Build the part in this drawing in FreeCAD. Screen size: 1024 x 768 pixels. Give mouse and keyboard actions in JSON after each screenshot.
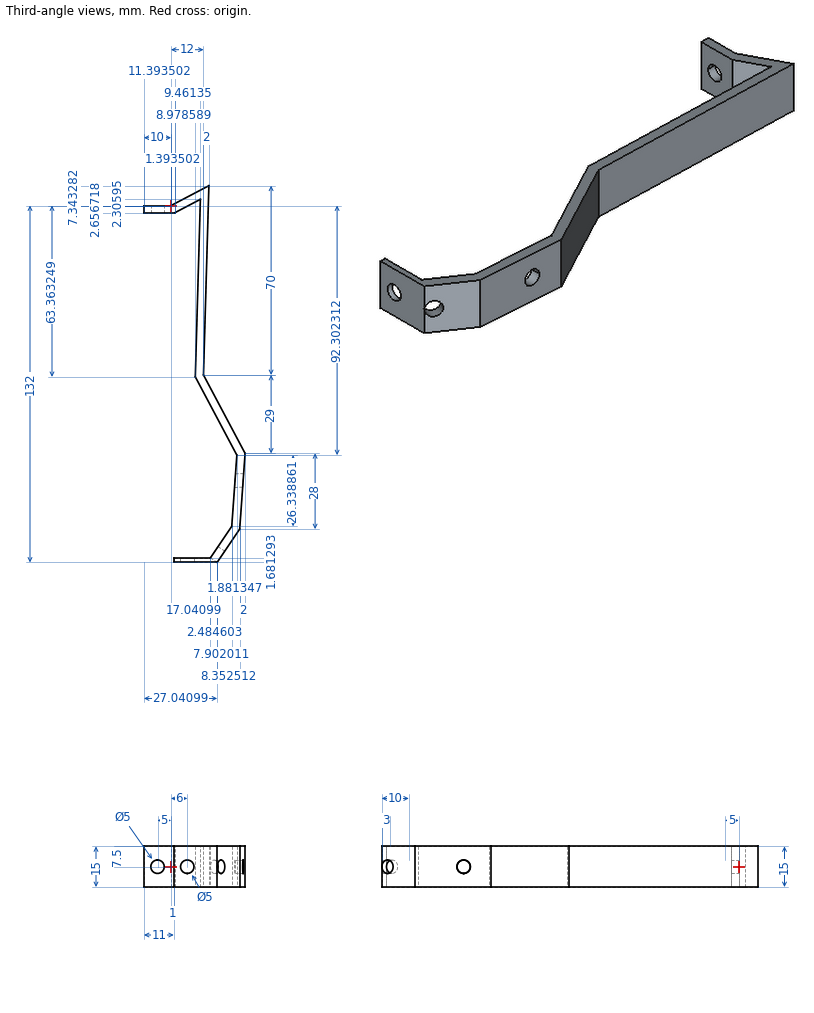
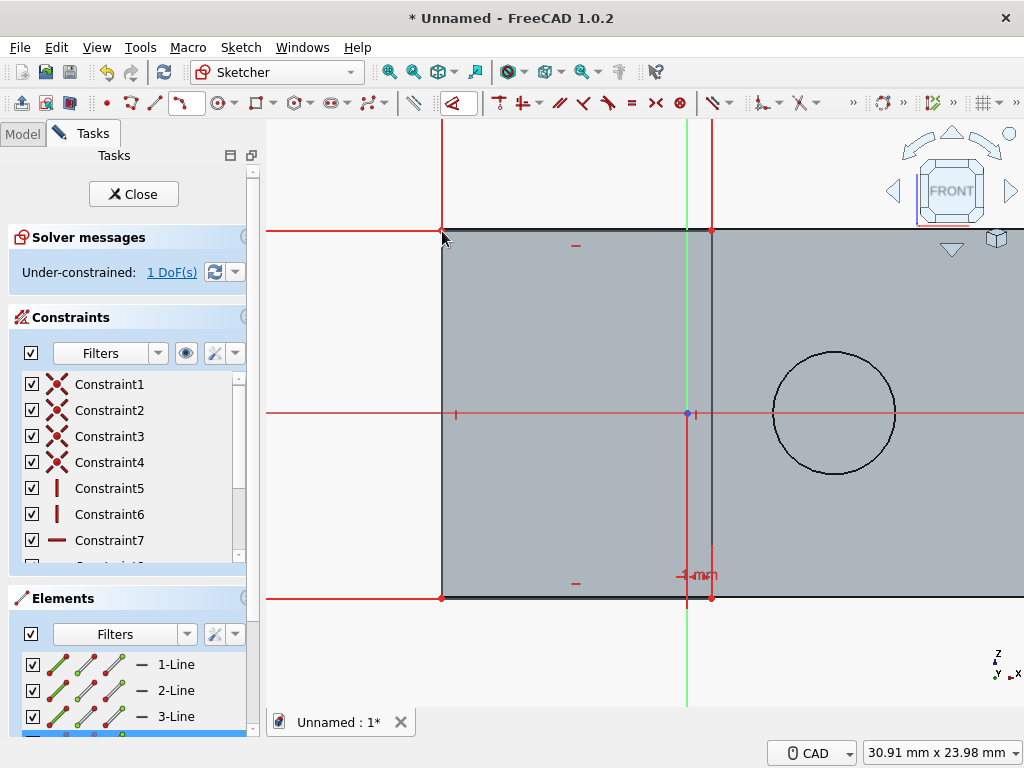
{"action": "key", "text": "i"}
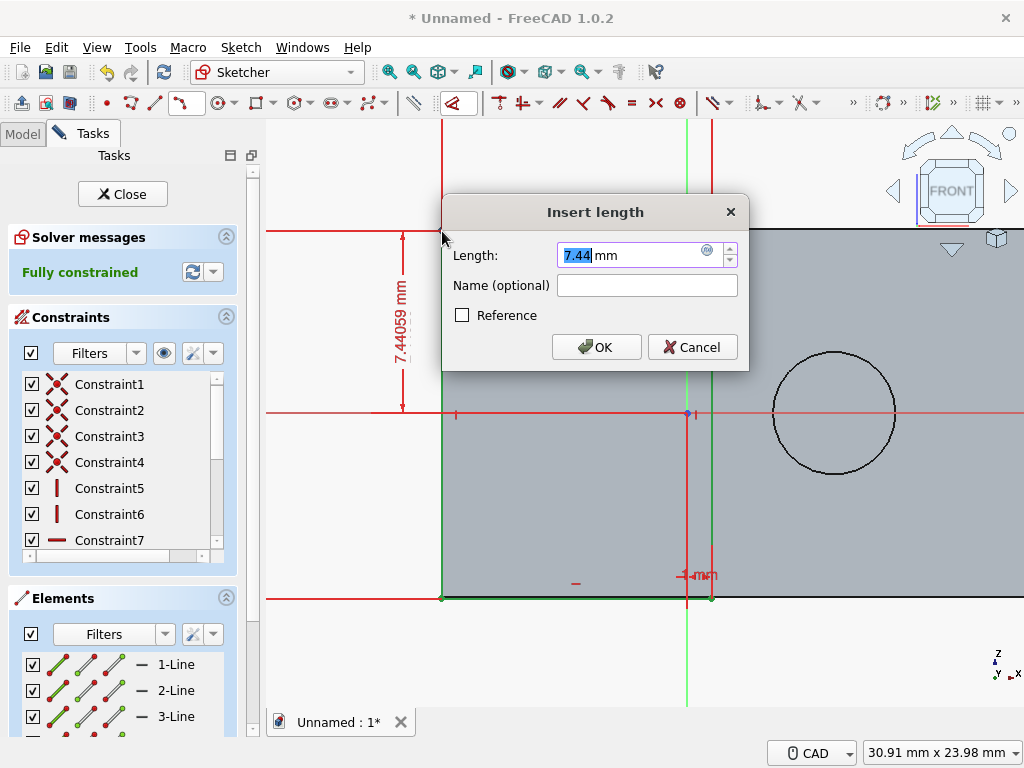
{"action": "type", "text": "7.5"}
{"action": "key", "text": "Return"}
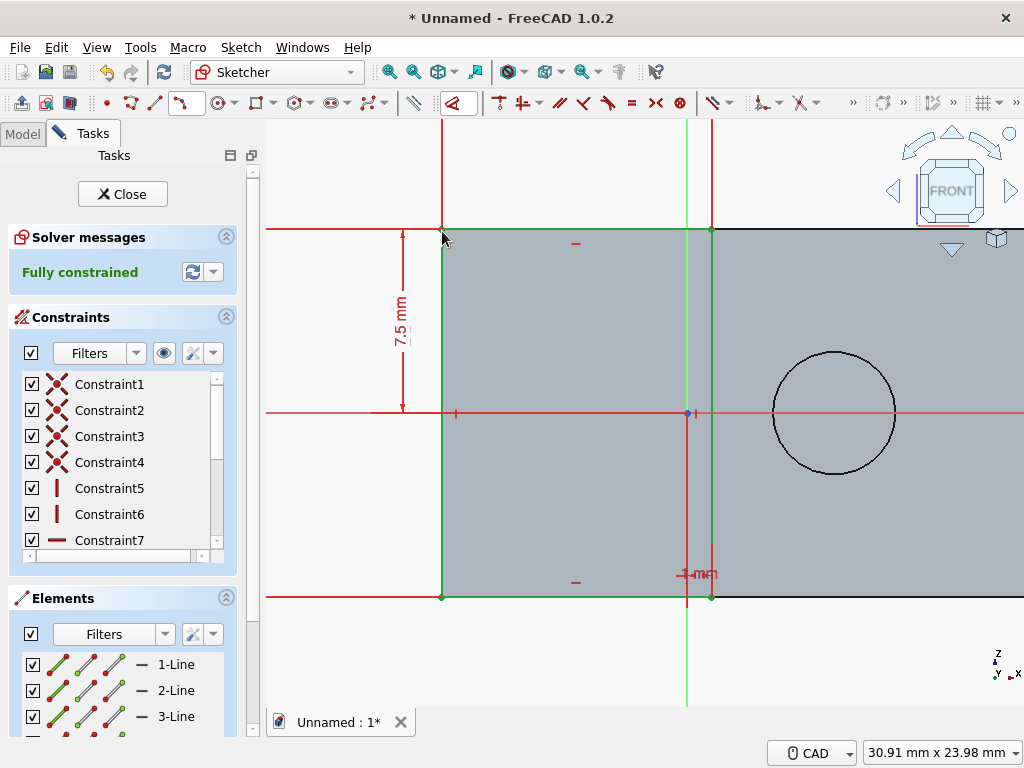
{"action": "left_click", "coordinate": [123, 194]}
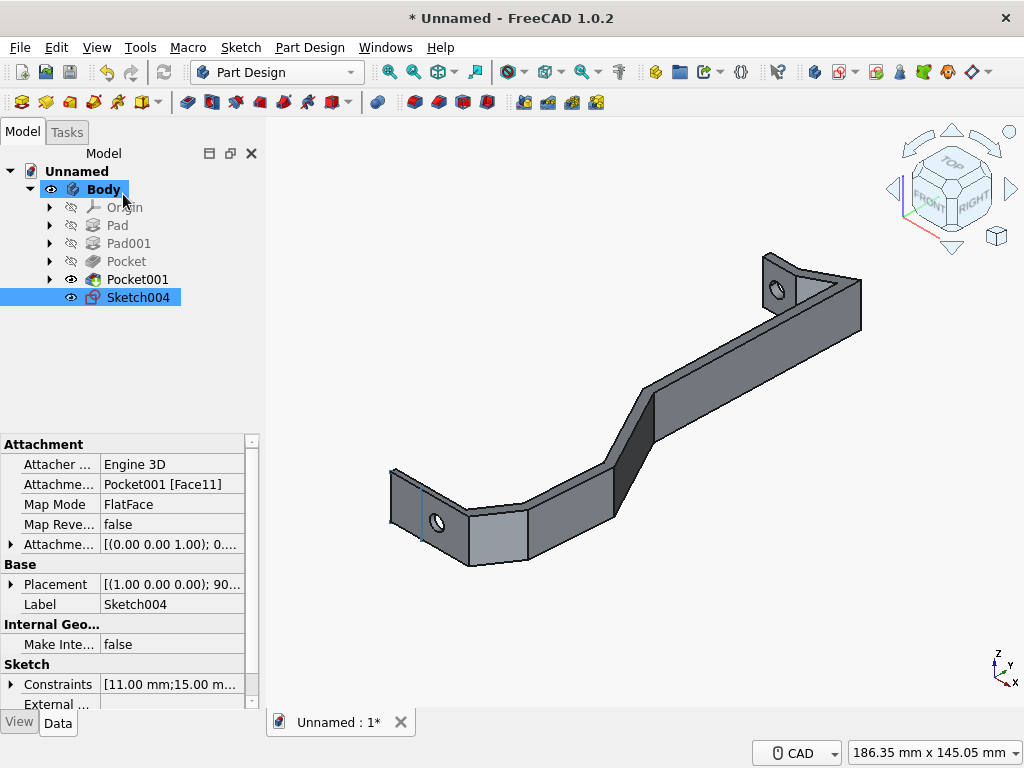
{"action": "left_click", "coordinate": [188, 102]}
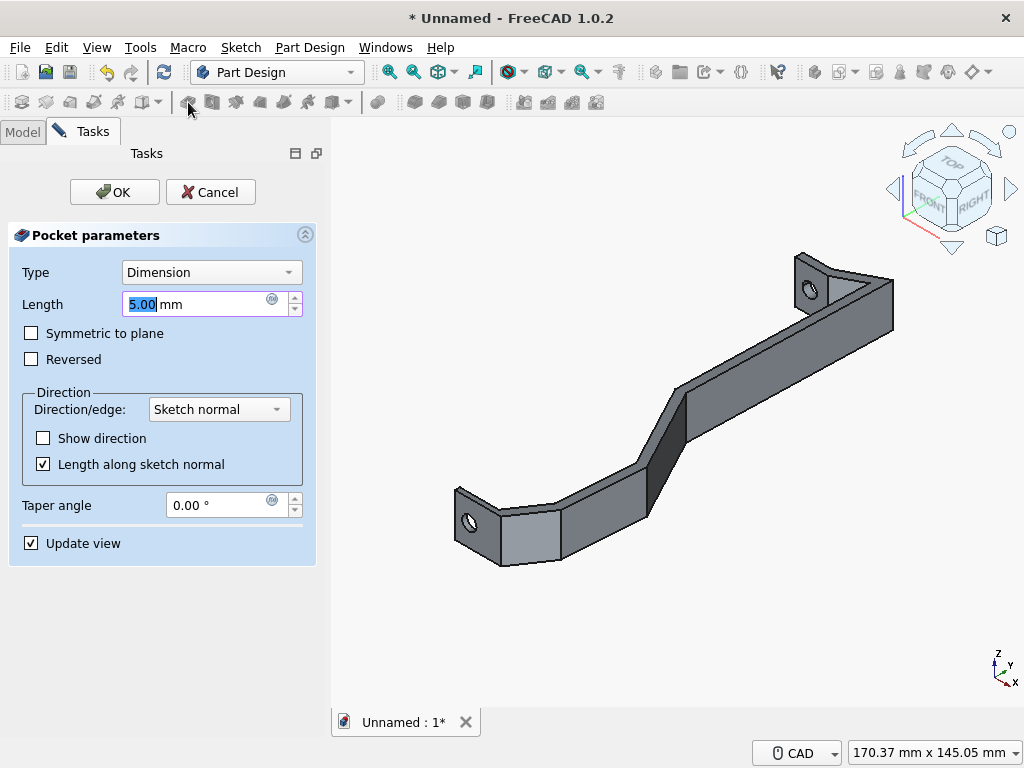
{"action": "type", "text": "3"}
{"action": "key", "text": "Tab"}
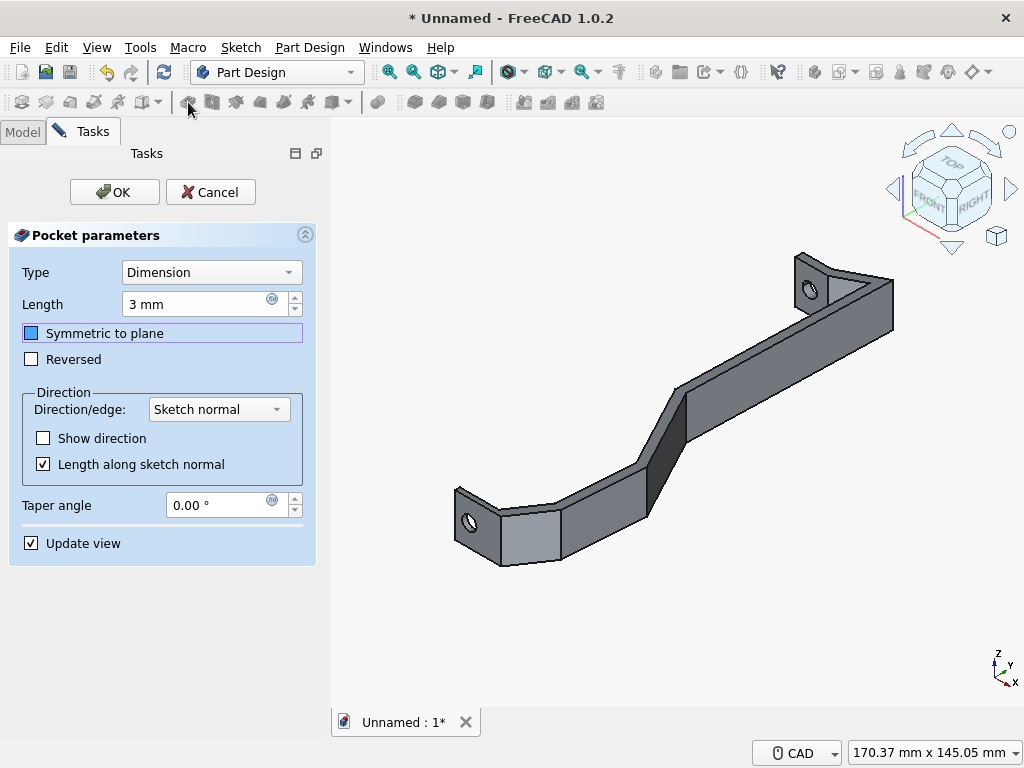
{"action": "left_click", "coordinate": [115, 192]}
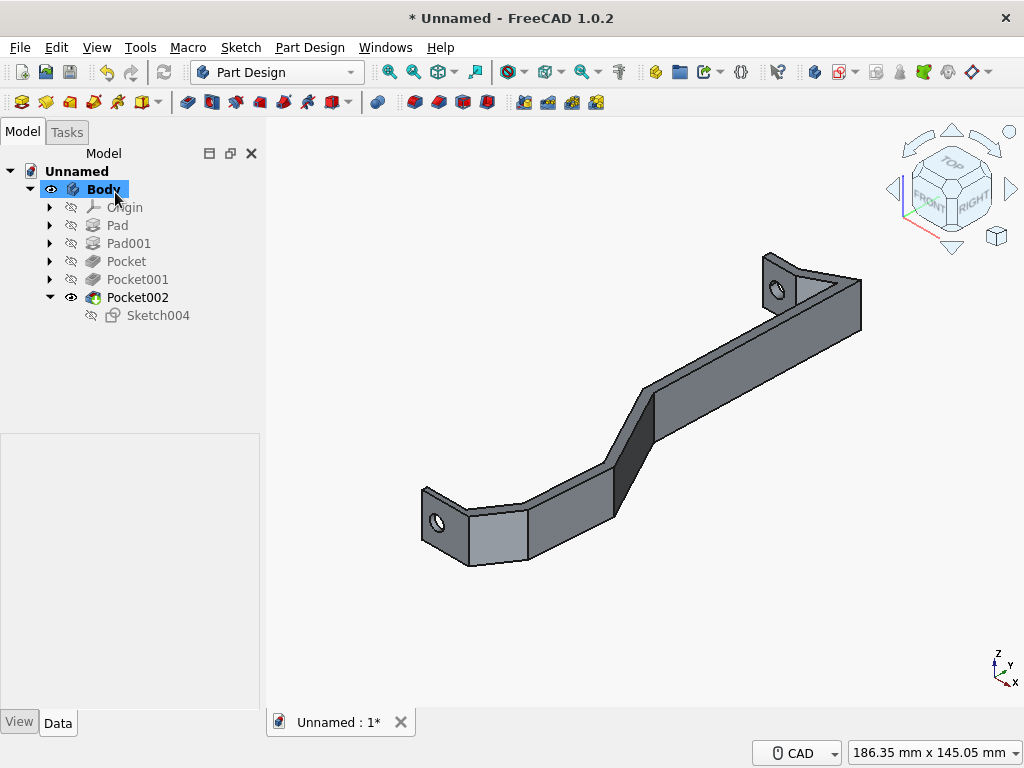
{"action": "left_click", "coordinate": [584, 506]}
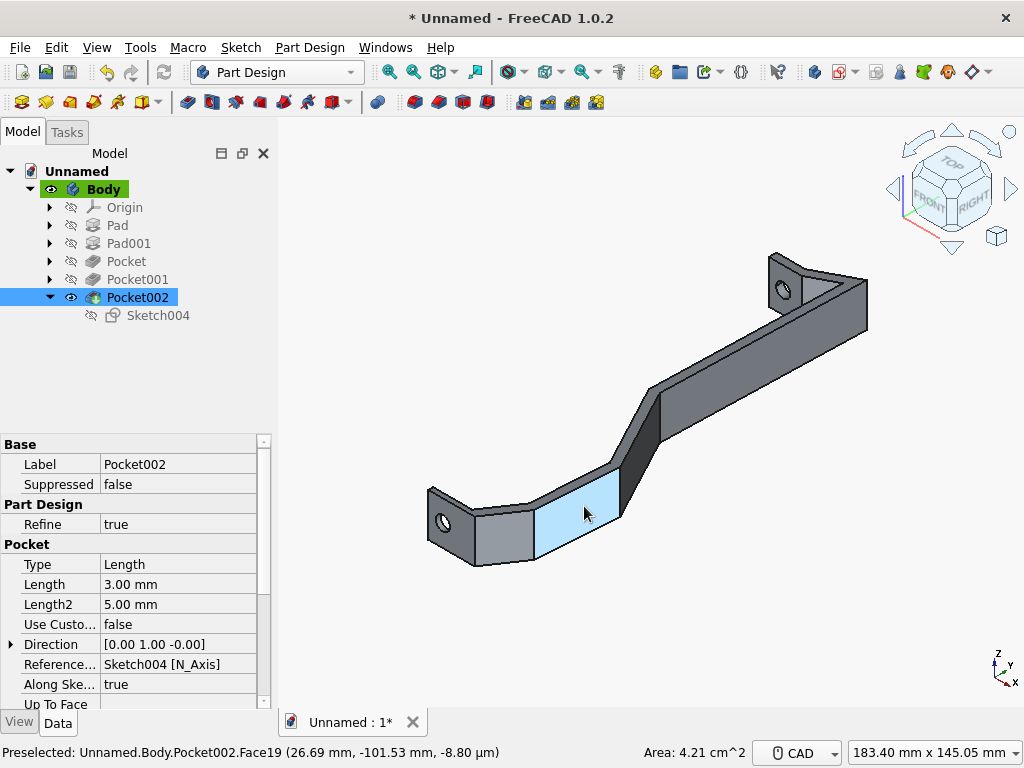
{"action": "left_click", "coordinate": [840, 72]}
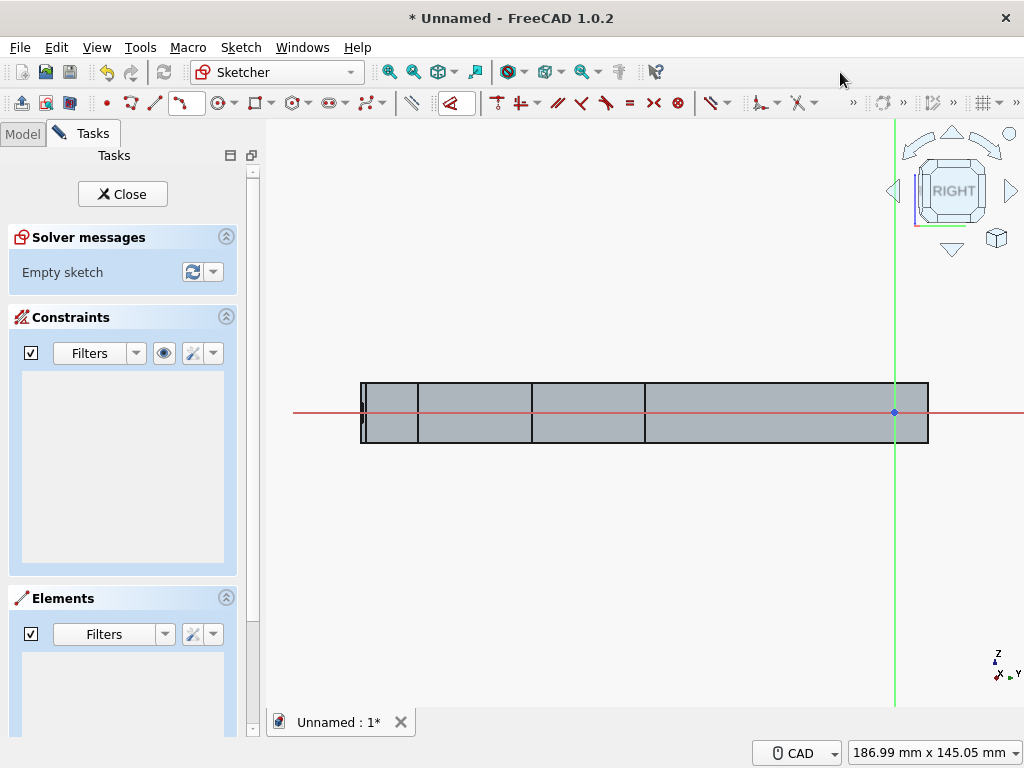
{"action": "scroll", "coordinate": [444, 413], "scroll_direction": "up", "scroll_amount": 9}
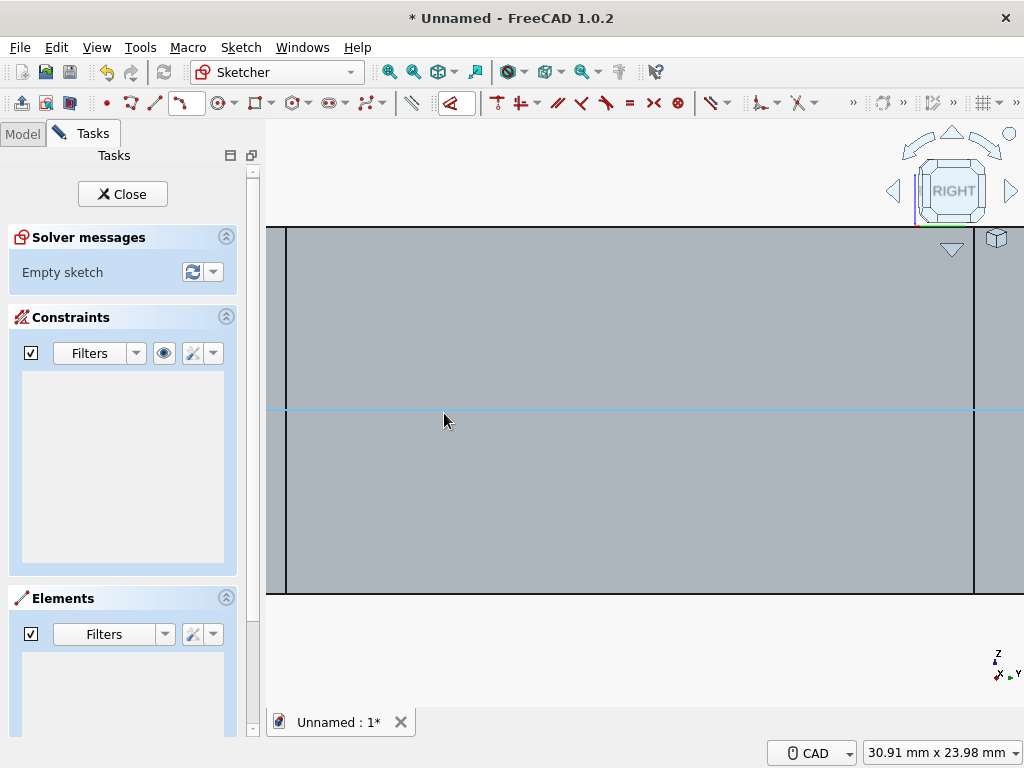
{"action": "left_click", "coordinate": [218, 104]}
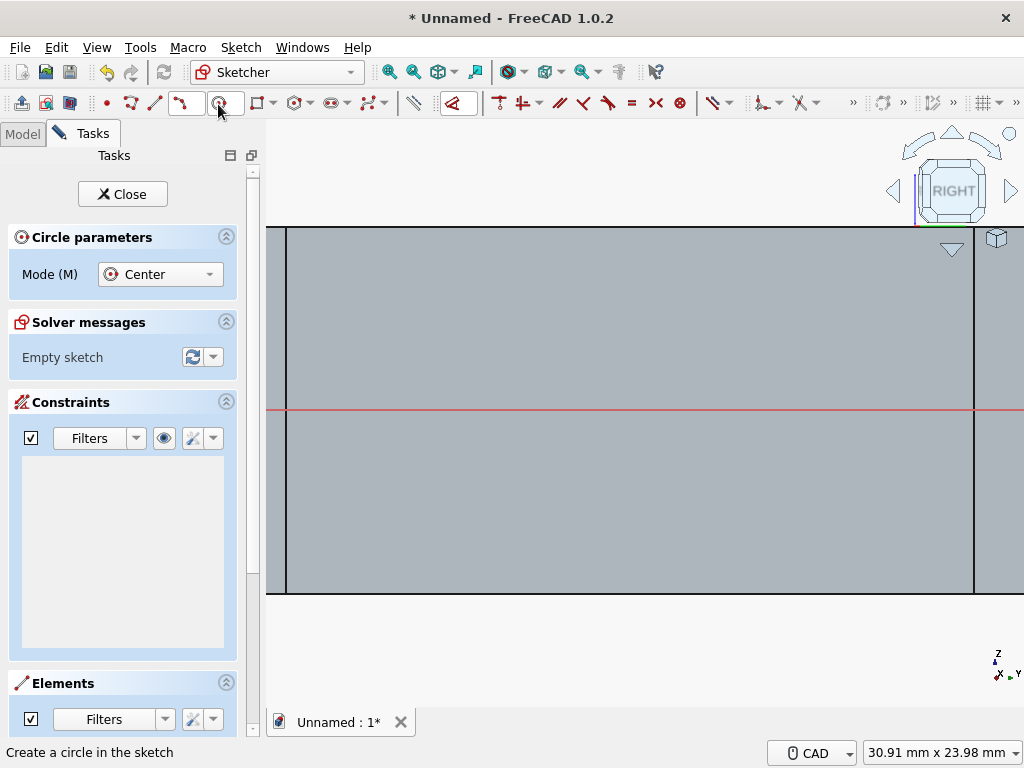
{"action": "left_click", "coordinate": [727, 410]}
{"action": "mouse_move", "coordinate": [770, 367]}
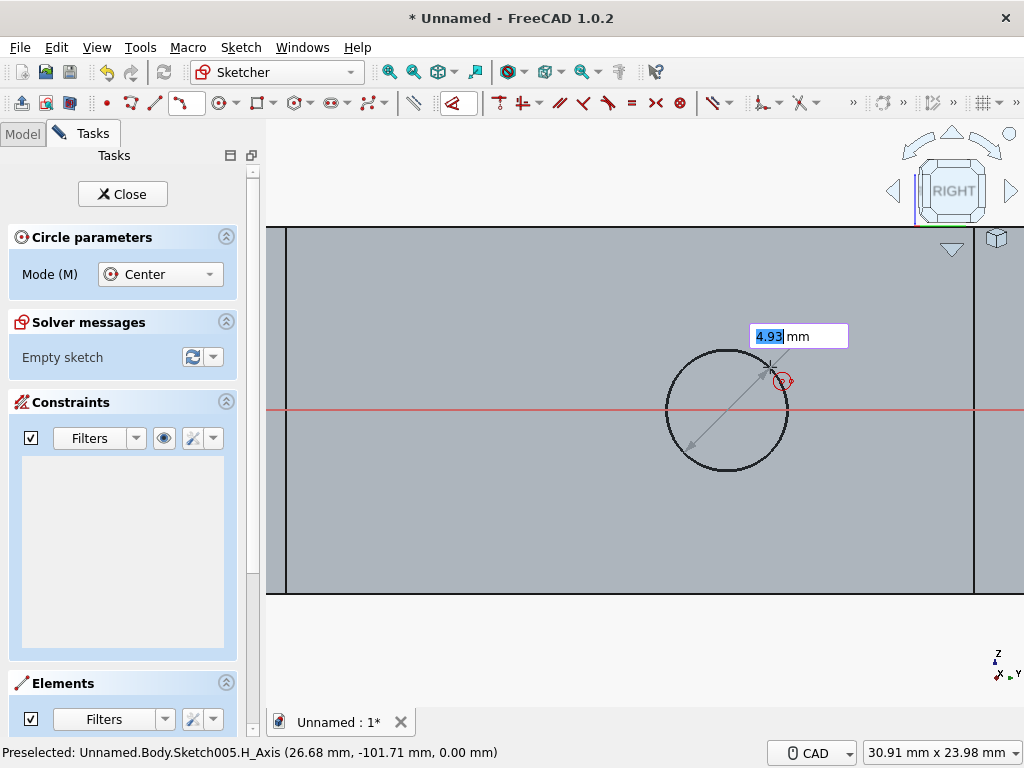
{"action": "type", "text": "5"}
{"action": "key", "text": "Return"}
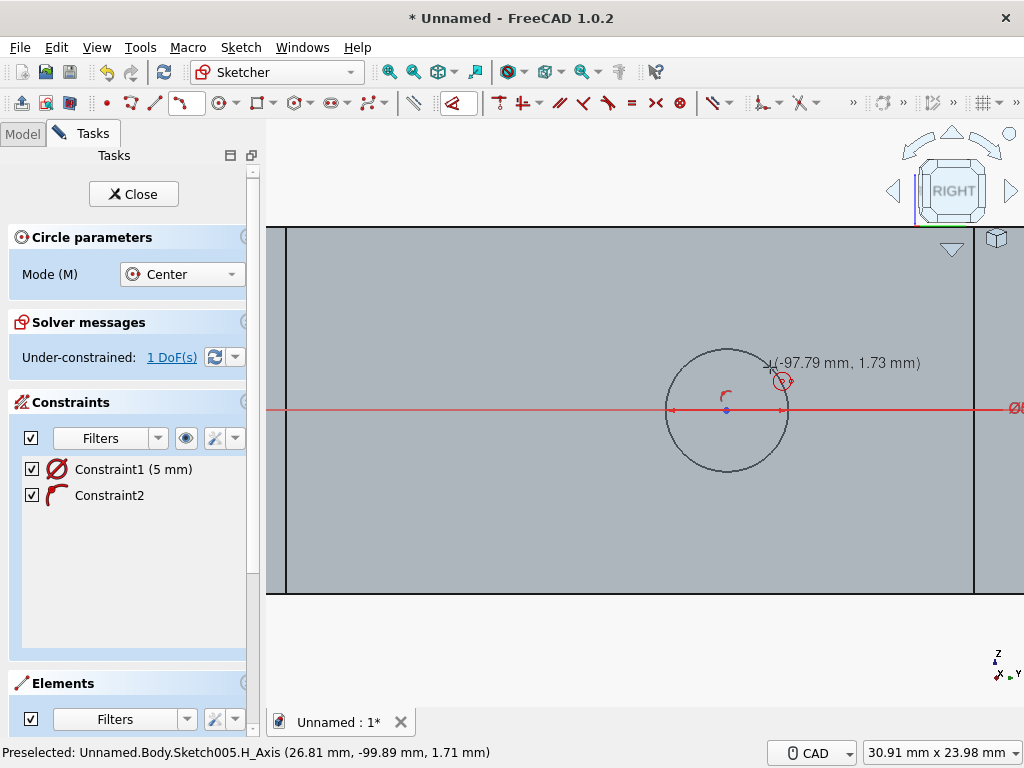
{"action": "left_click", "coordinate": [156, 104]}